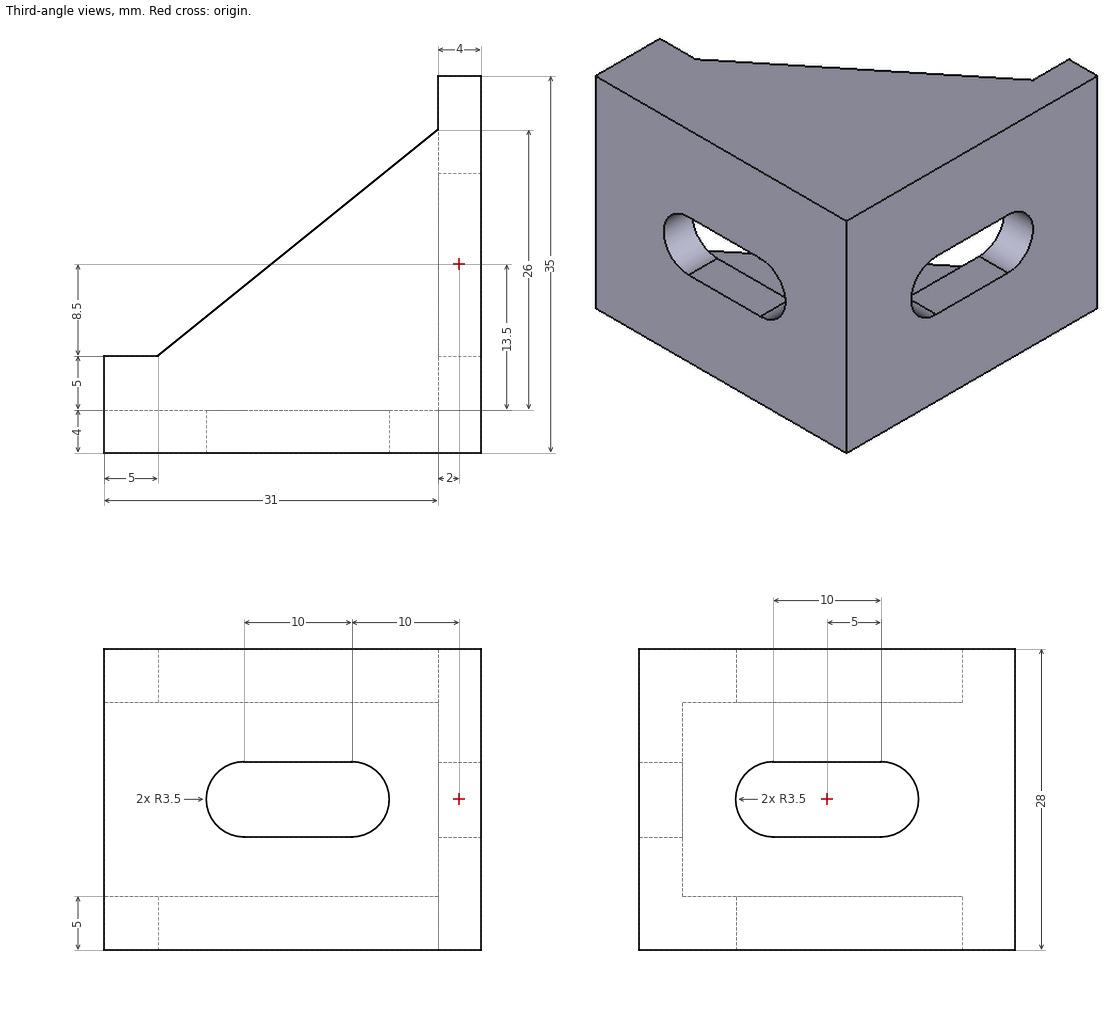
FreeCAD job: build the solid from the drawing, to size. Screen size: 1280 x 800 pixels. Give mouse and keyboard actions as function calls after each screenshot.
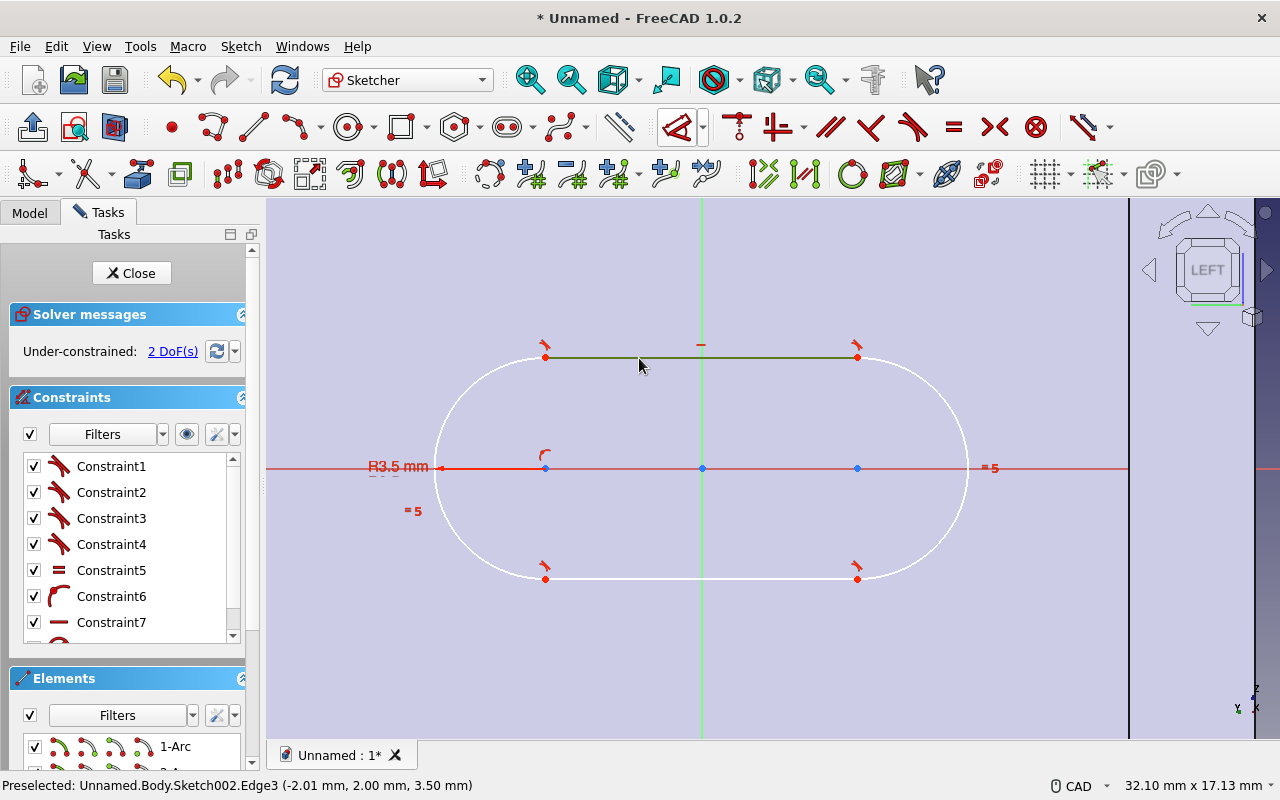
click(702, 128)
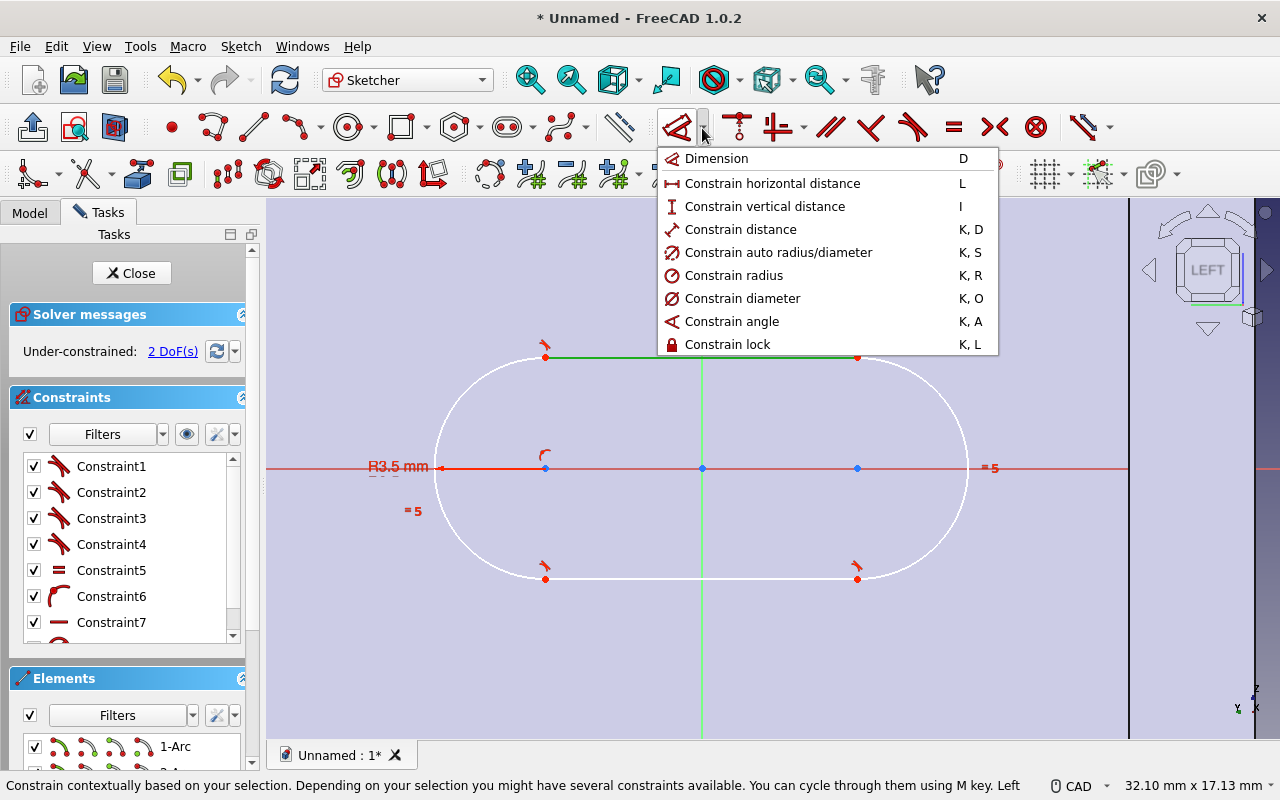
click(828, 184)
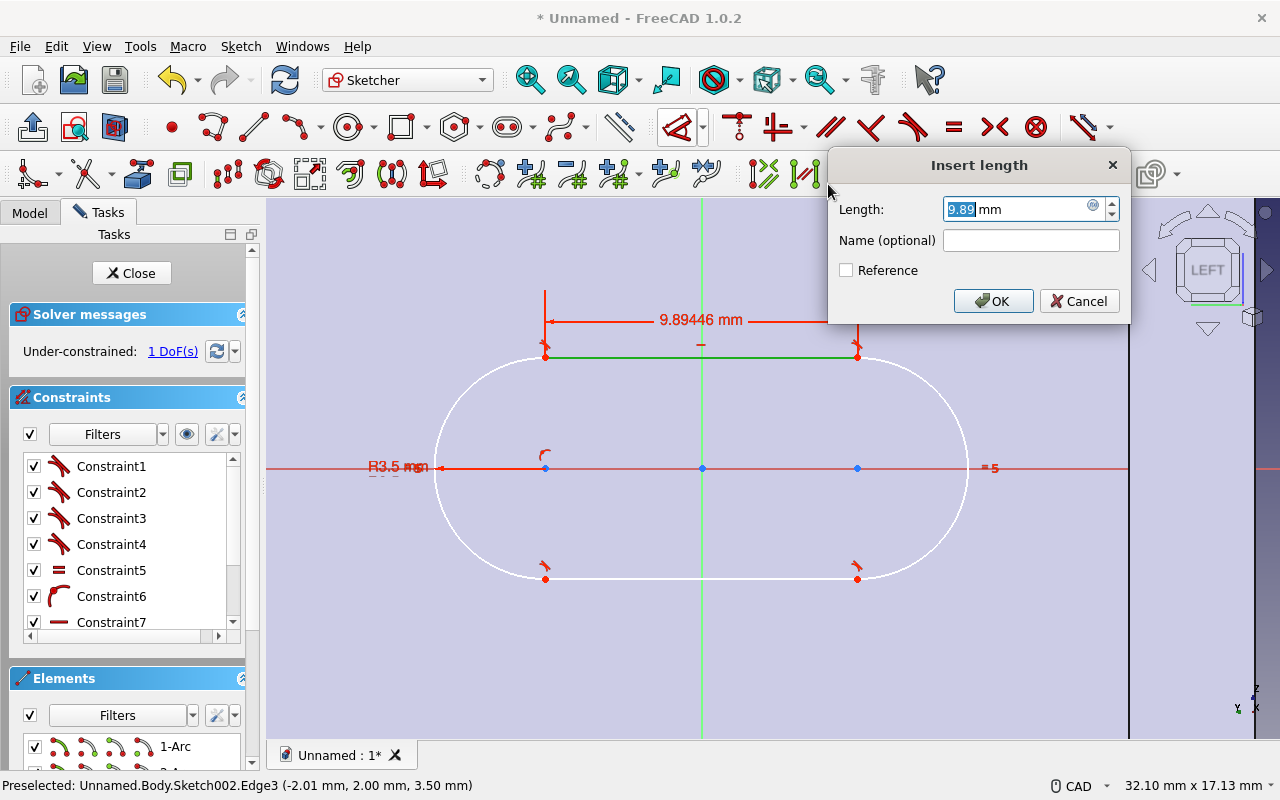
text(10)
key(Return)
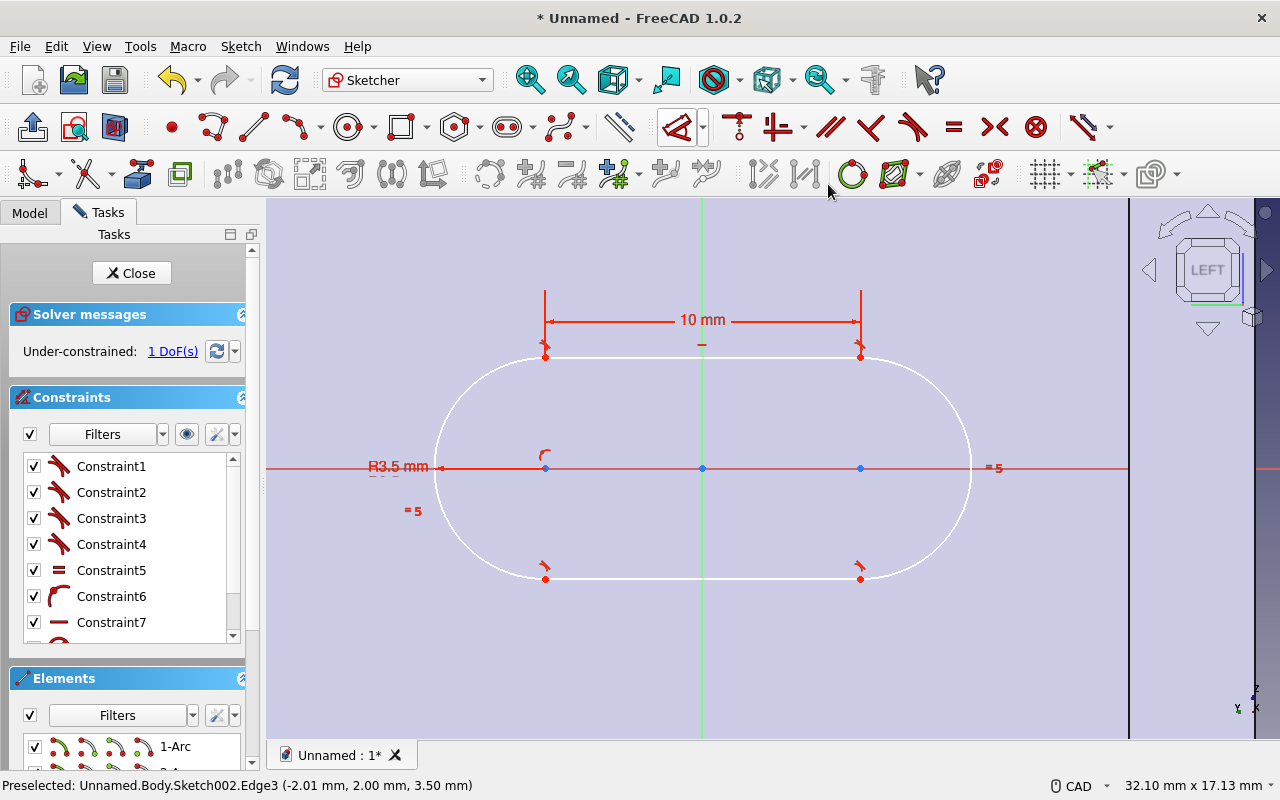
click(545, 358)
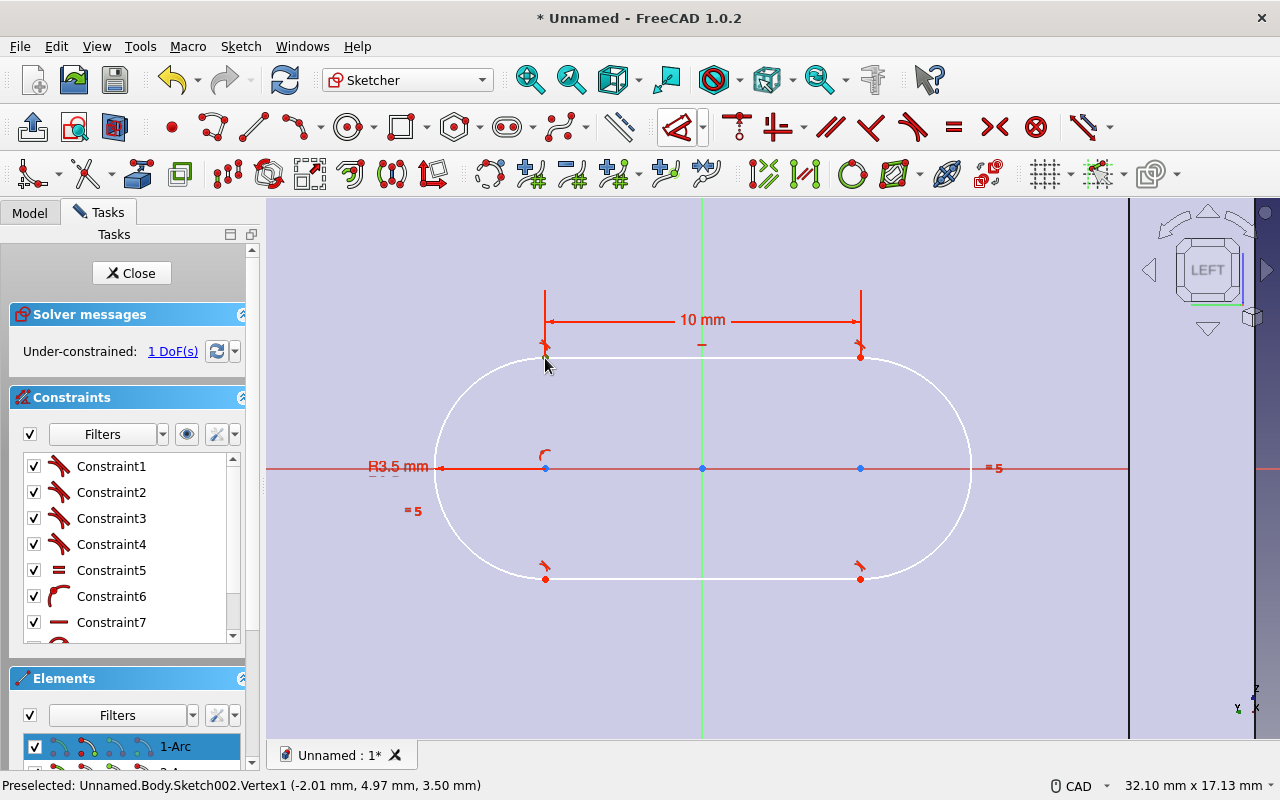
key(l)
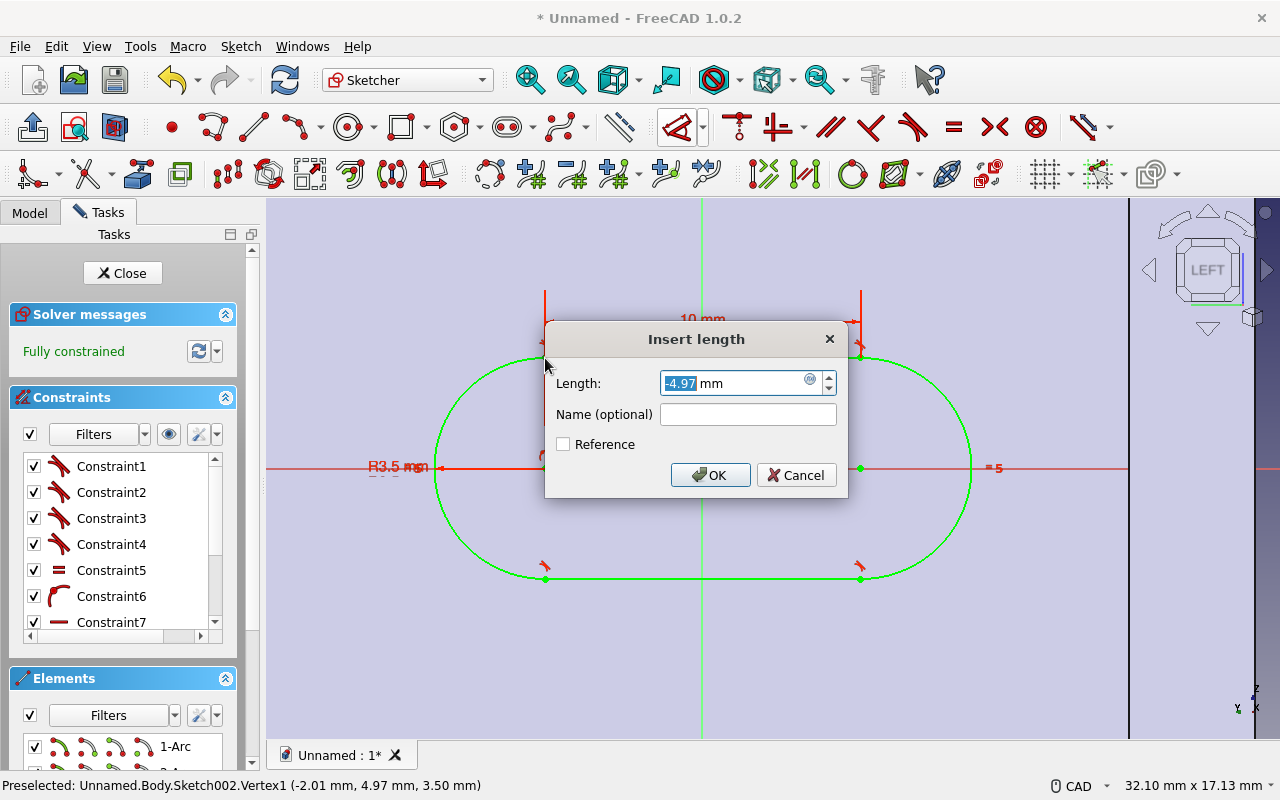
text(-5)
key(Return)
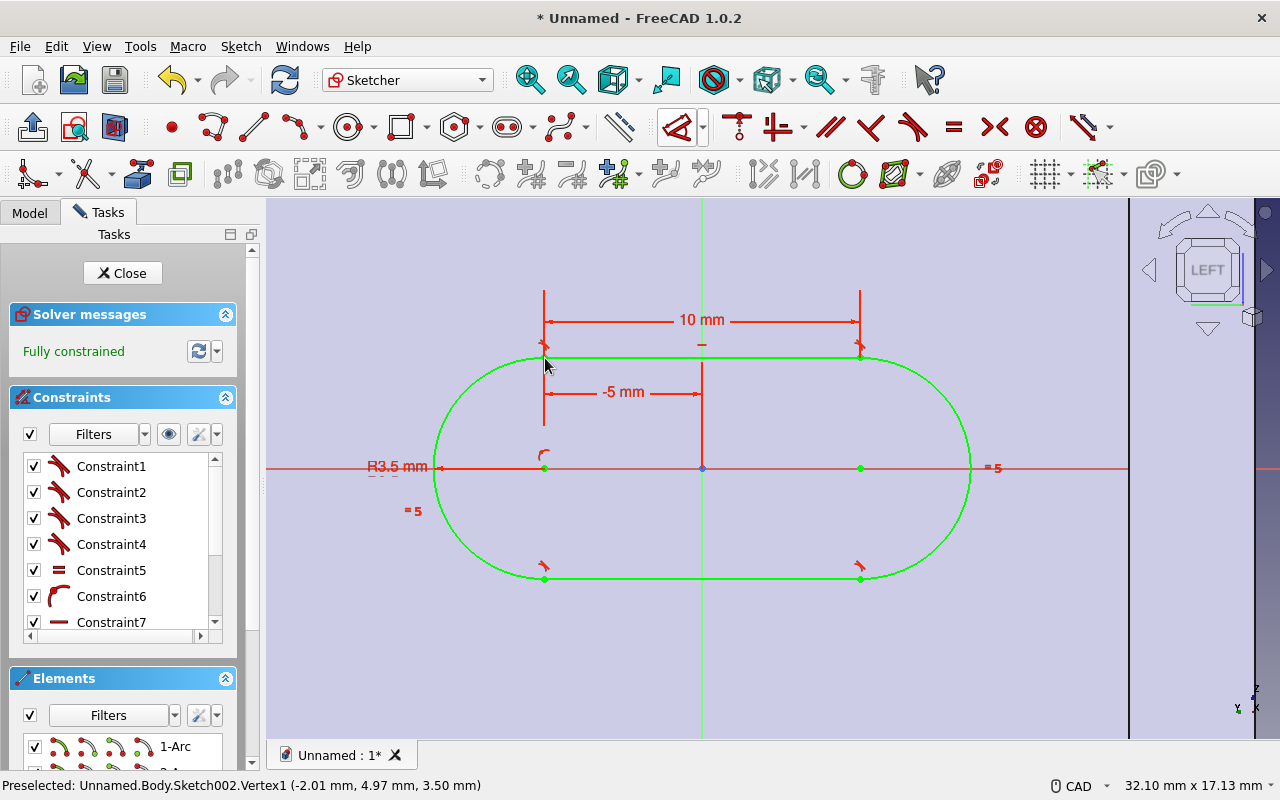
click(123, 273)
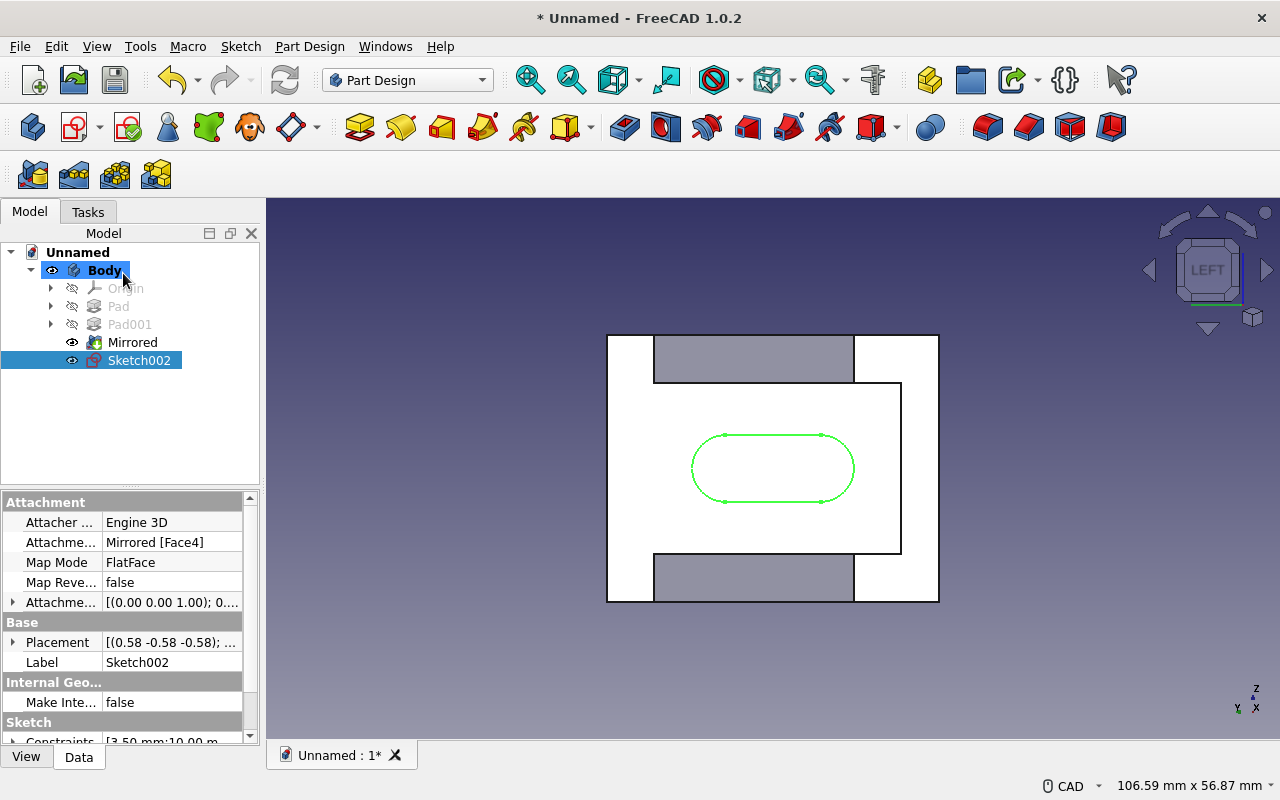
click(625, 128)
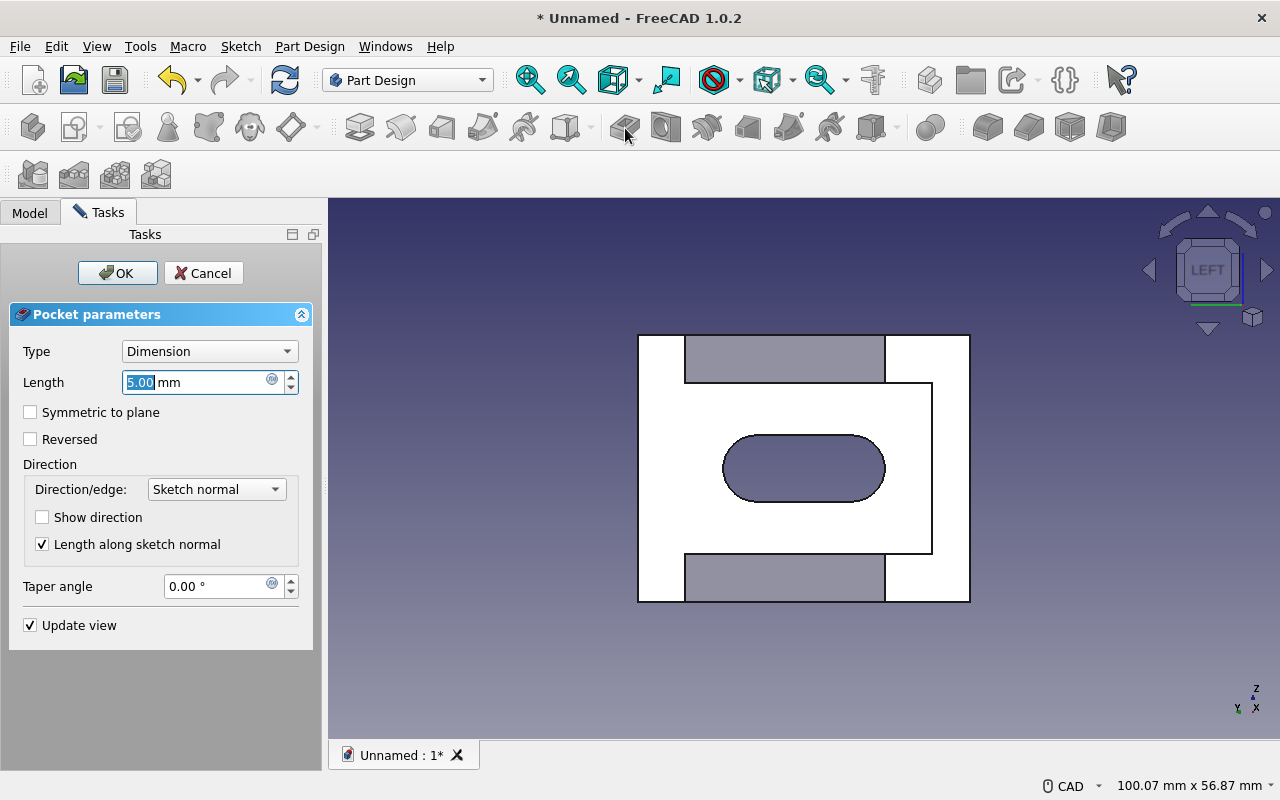
text(5)
key(Tab)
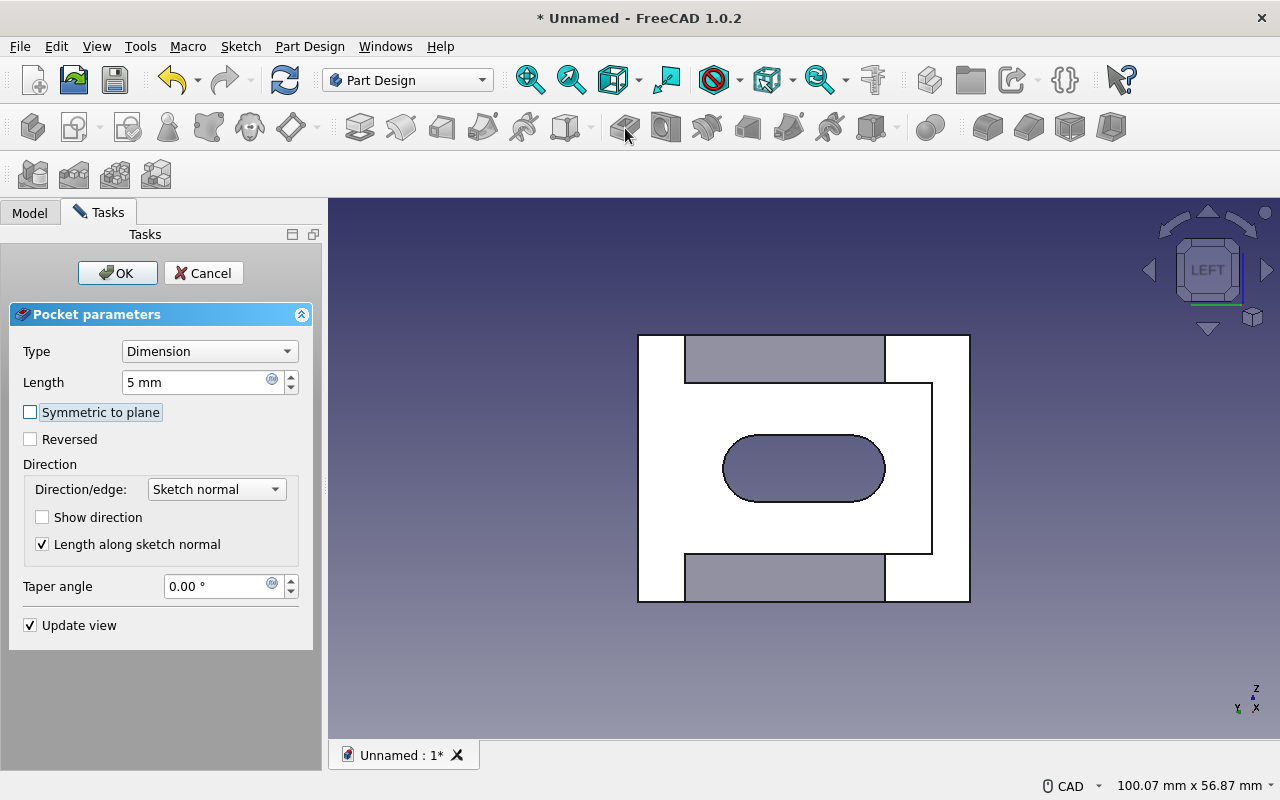
click(118, 273)